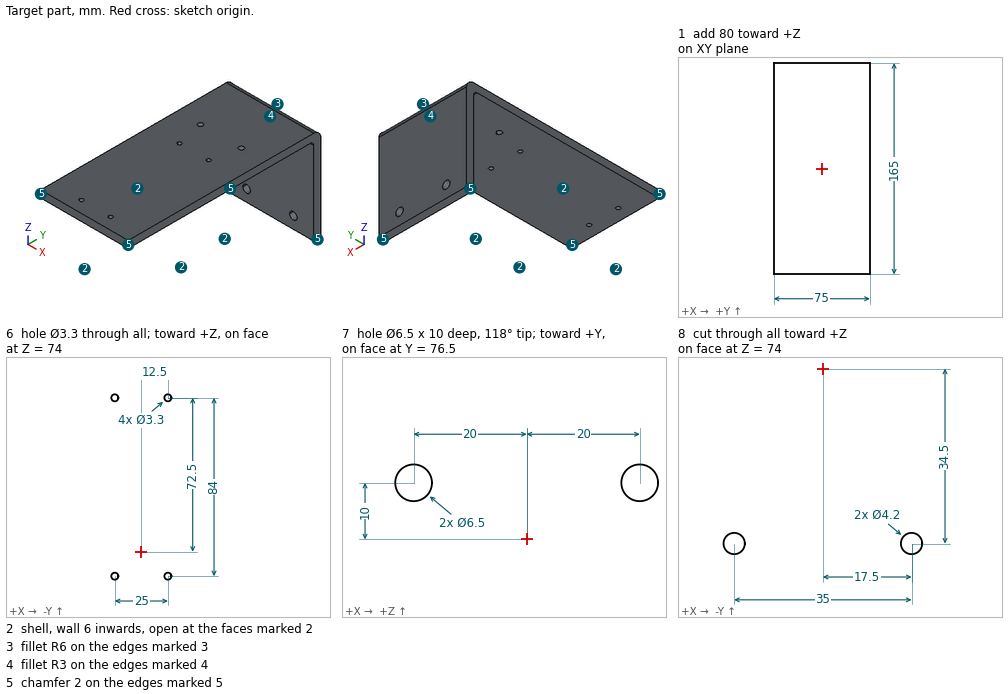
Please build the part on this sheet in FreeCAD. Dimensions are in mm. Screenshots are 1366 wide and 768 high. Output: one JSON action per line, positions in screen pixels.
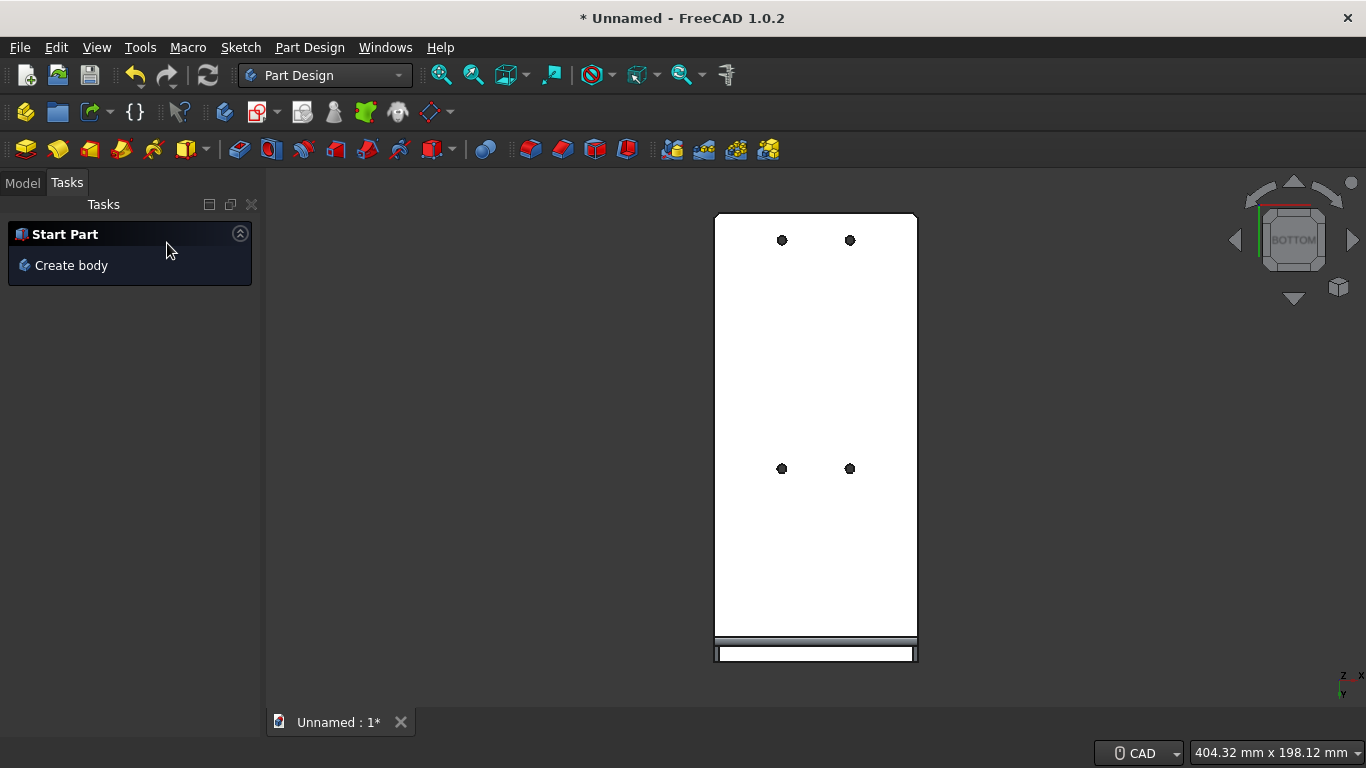
{"action": "left_click", "coordinate": [816, 364]}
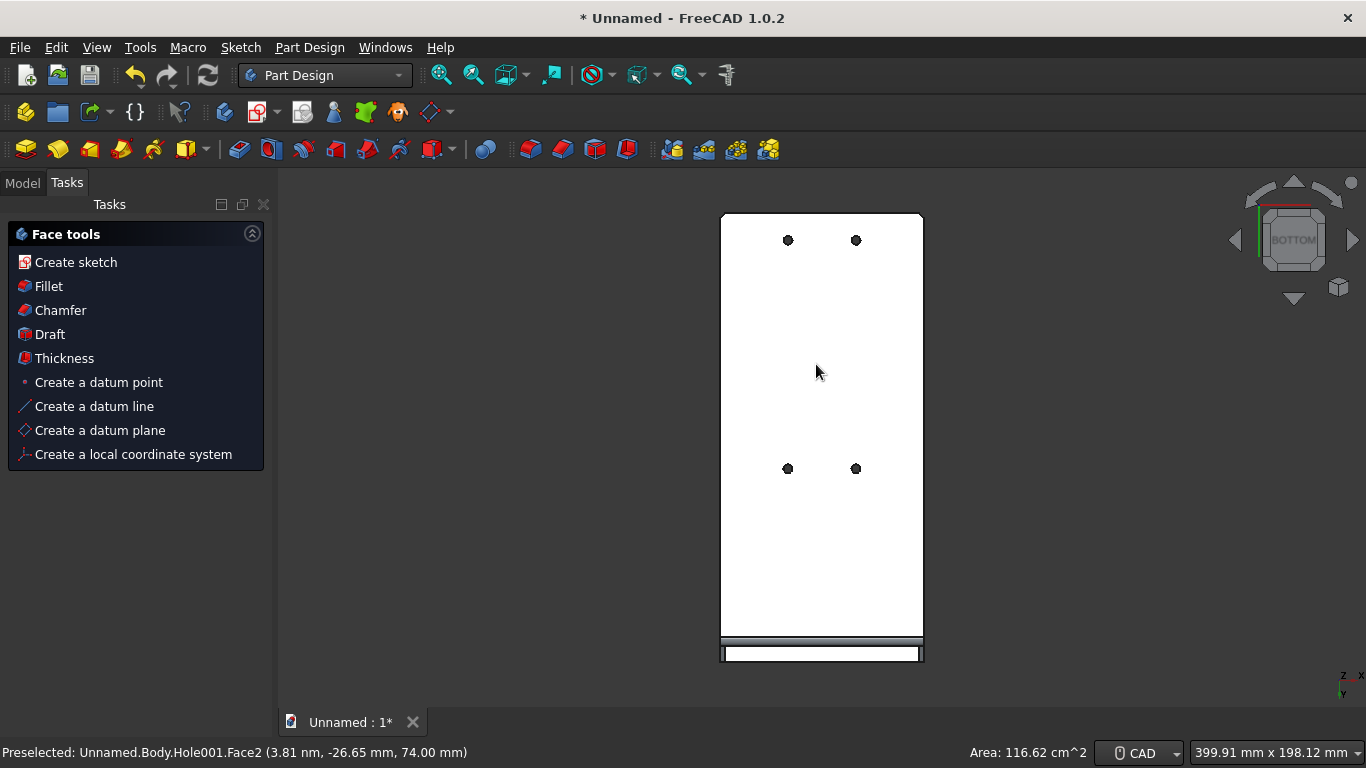
{"action": "left_click", "coordinate": [258, 112]}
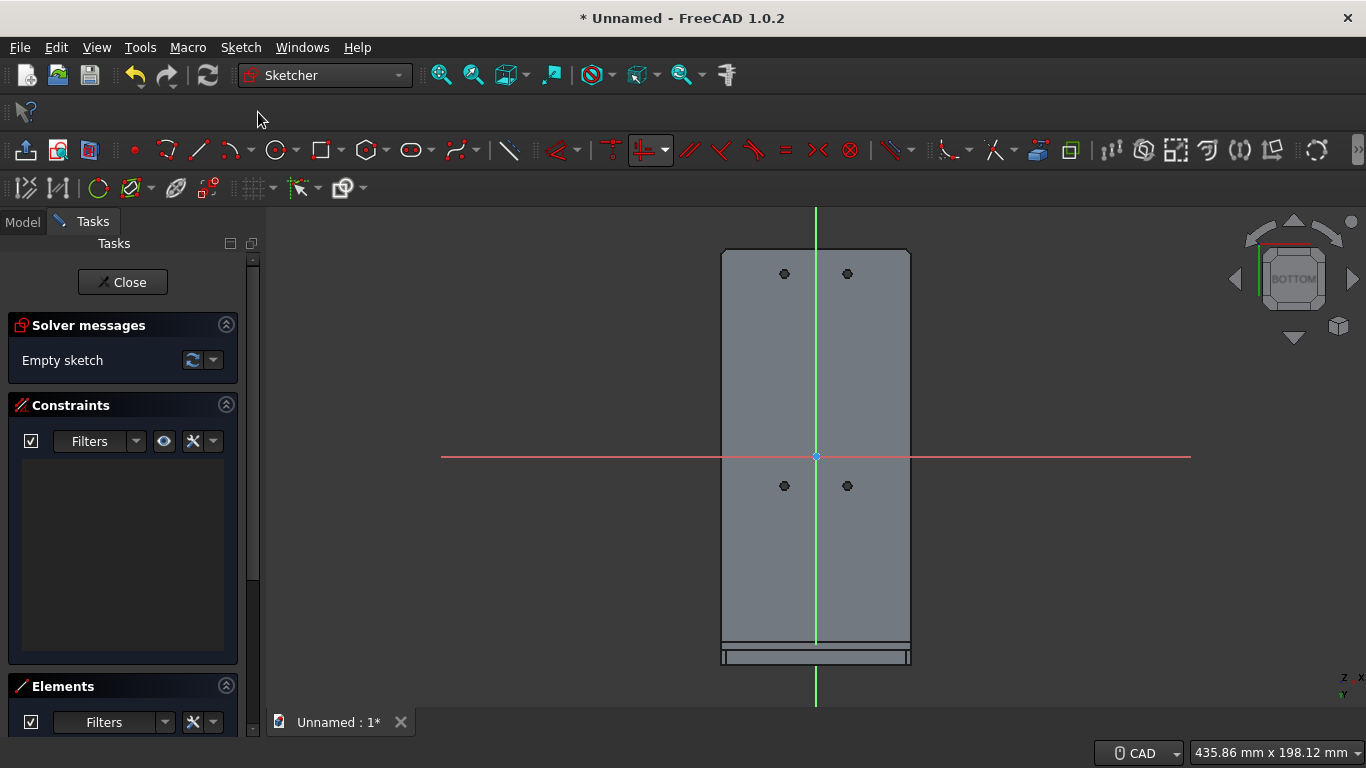
{"action": "left_click", "coordinate": [90, 150]}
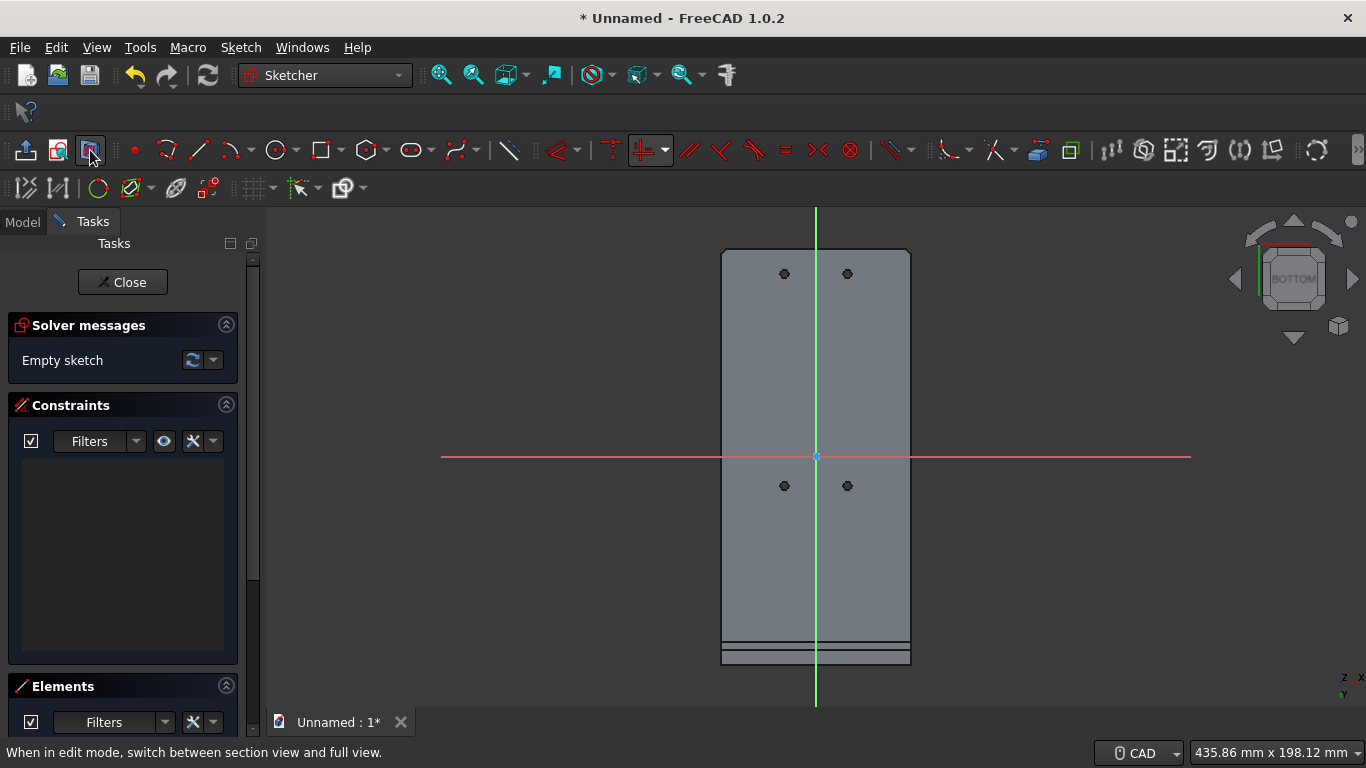
{"action": "scroll", "coordinate": [846, 523], "scroll_direction": "up", "scroll_amount": 6}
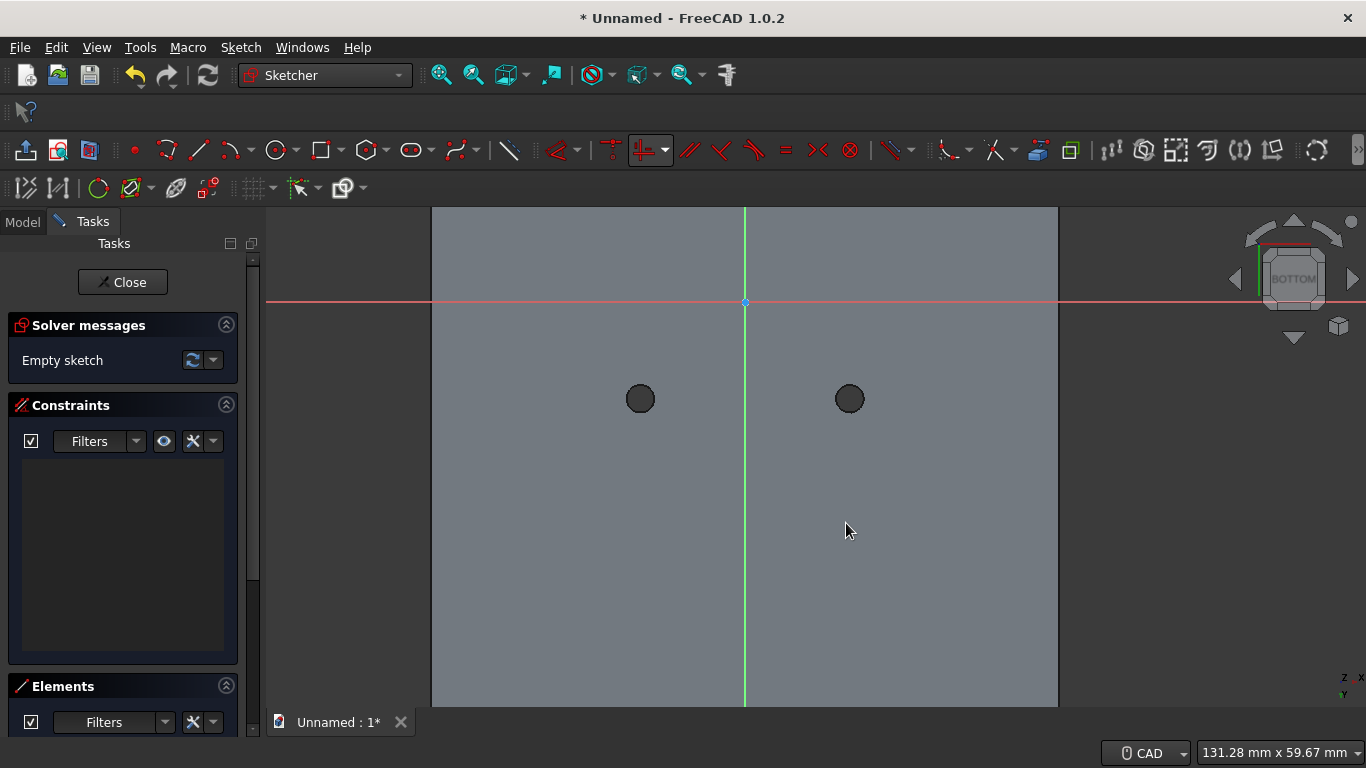
{"action": "left_click", "coordinate": [276, 150]}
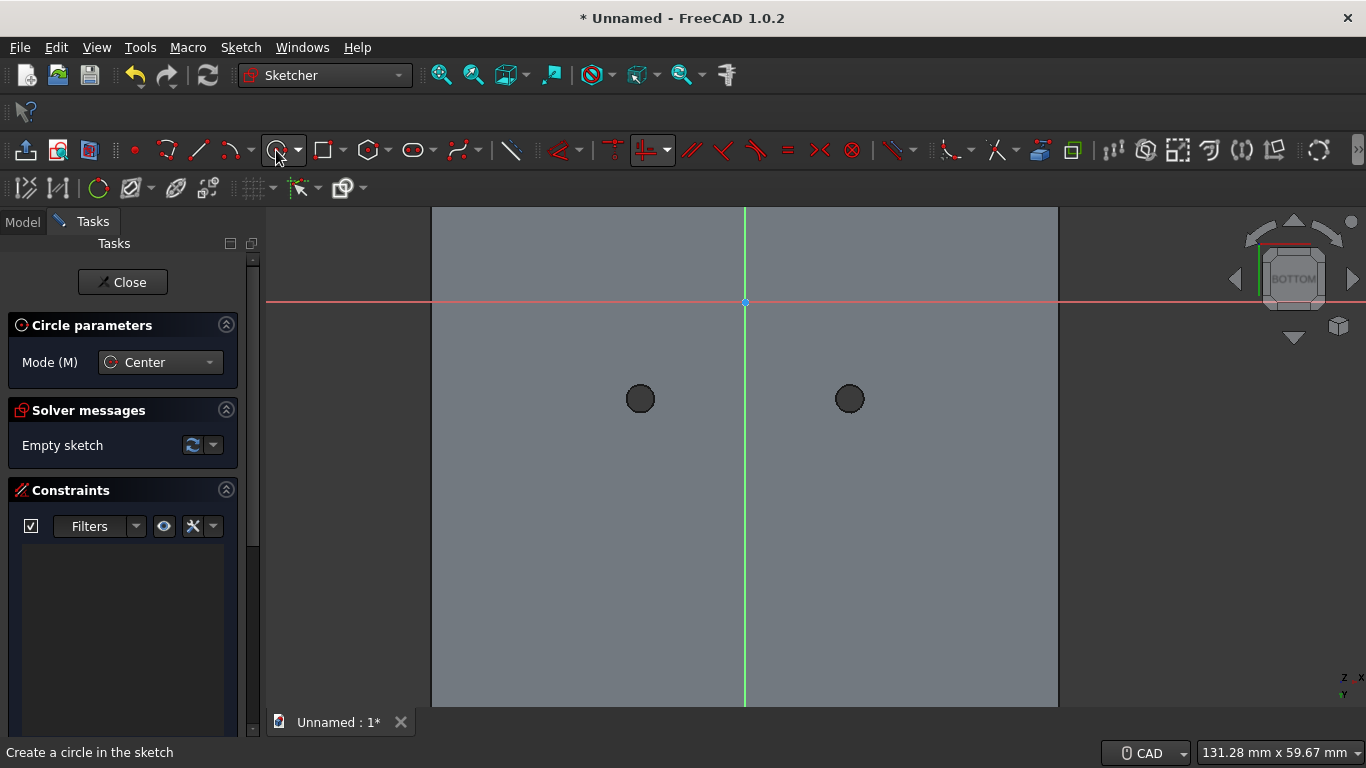
{"action": "scroll", "coordinate": [892, 591], "scroll_direction": "up", "scroll_amount": 2}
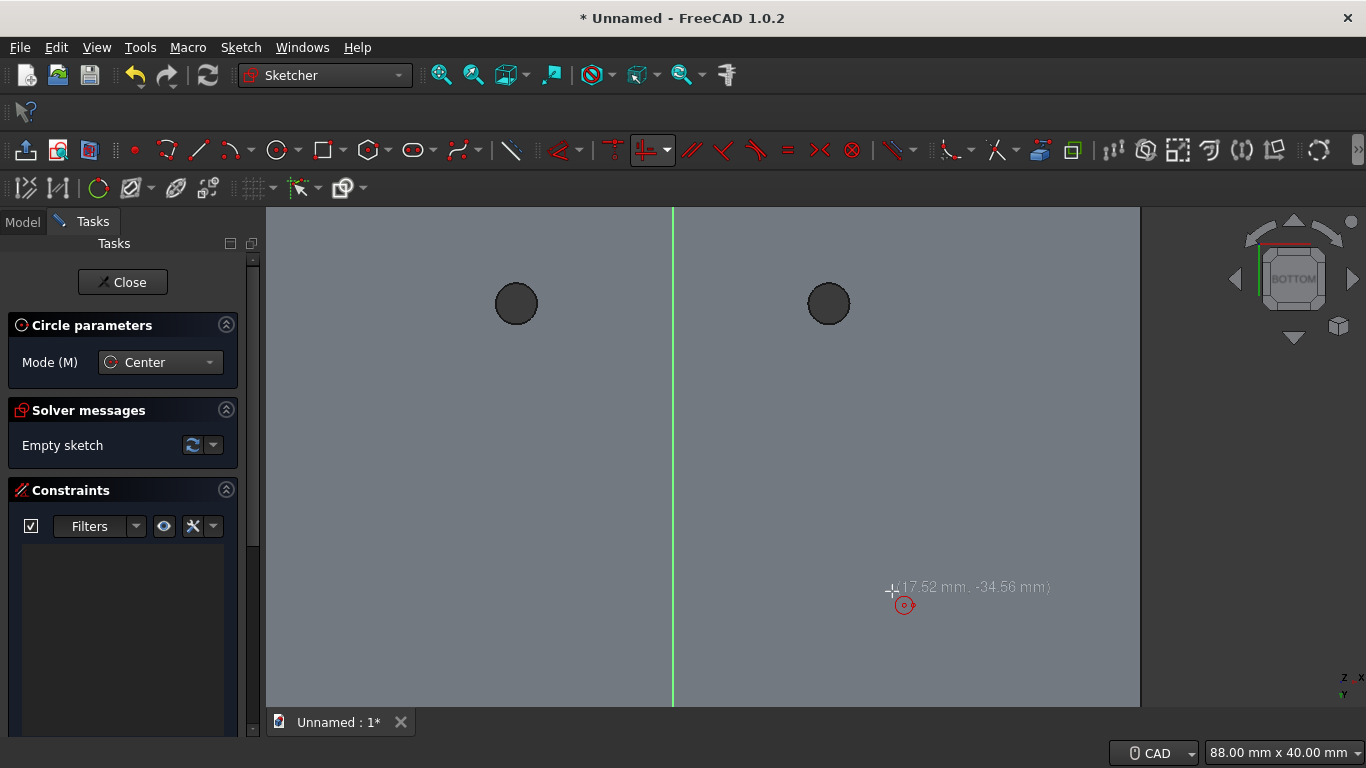
{"action": "left_click", "coordinate": [891, 591]}
{"action": "left_click", "coordinate": [910, 573]}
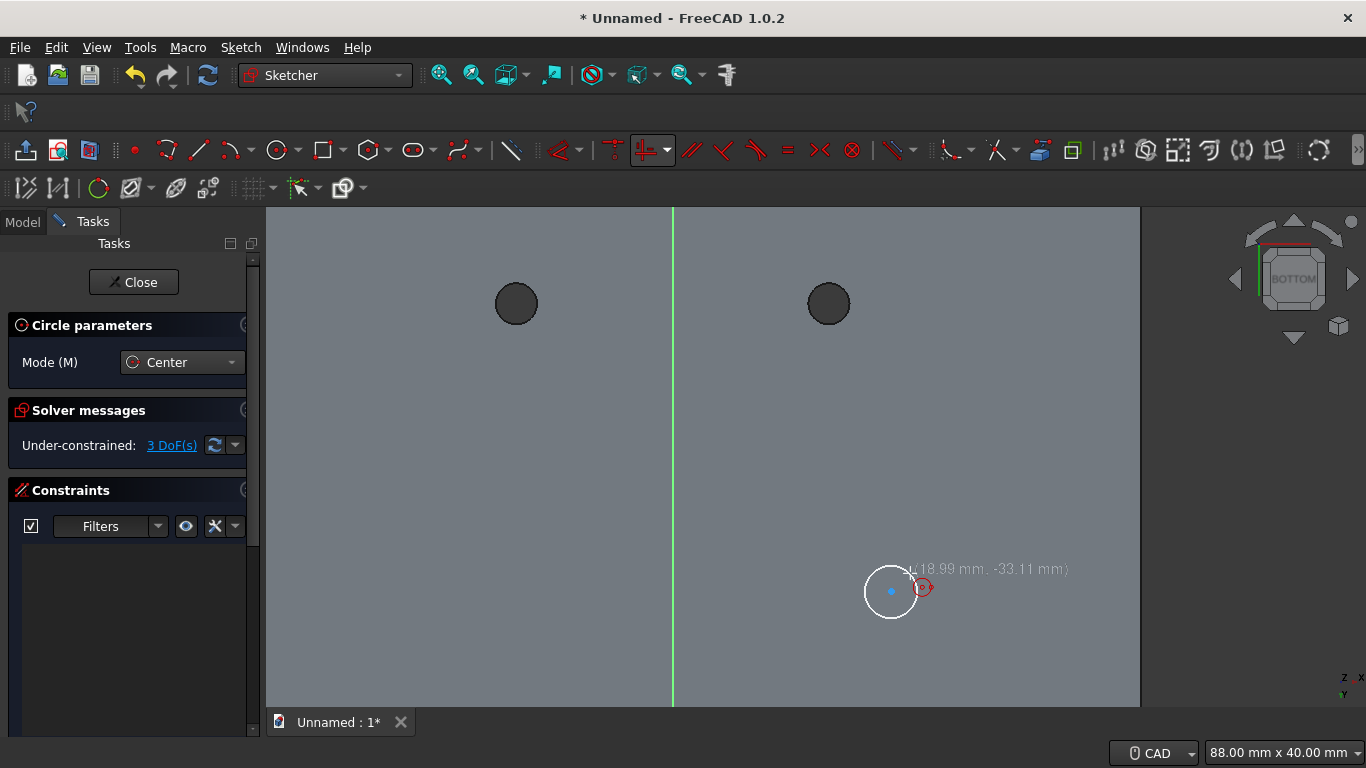
{"action": "left_click", "coordinate": [454, 591]}
{"action": "left_click", "coordinate": [472, 573]}
{"action": "key", "text": "Escape"}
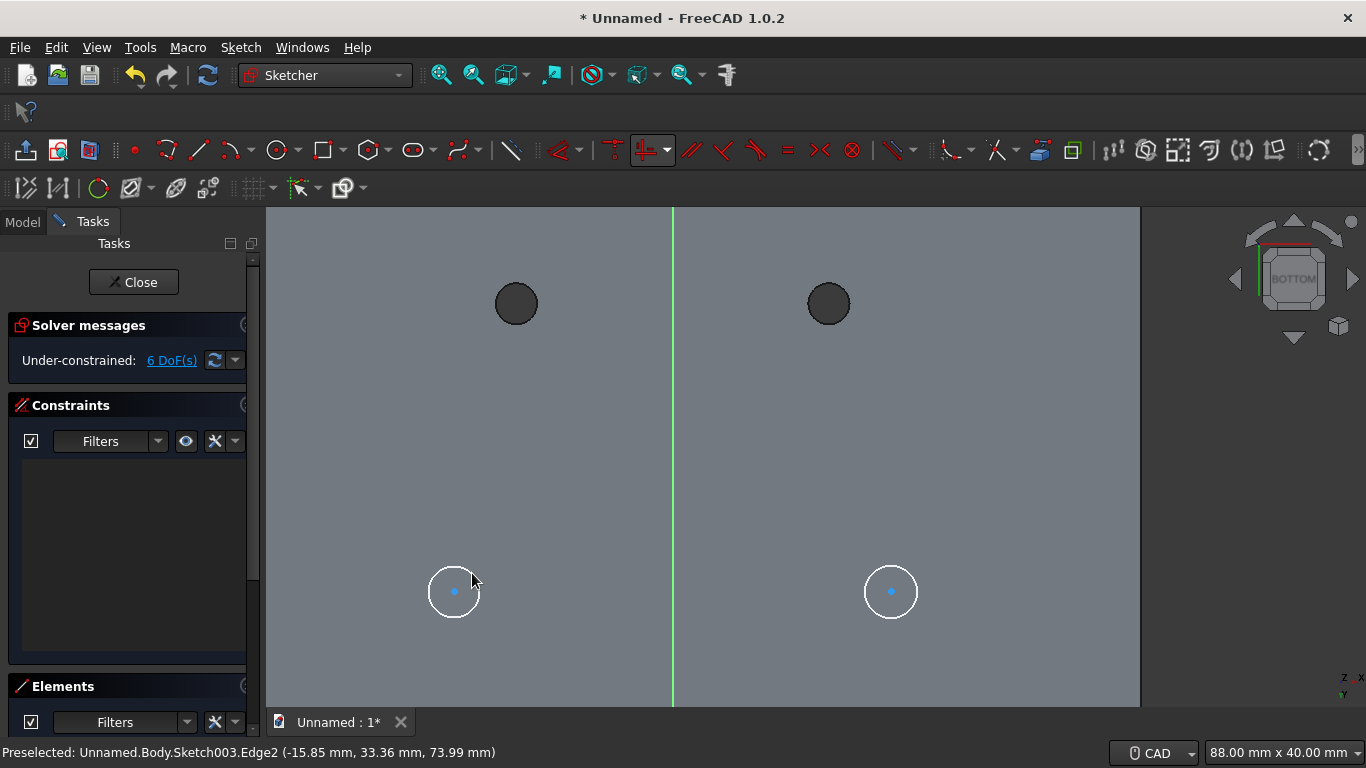
{"action": "left_click", "coordinate": [909, 573]}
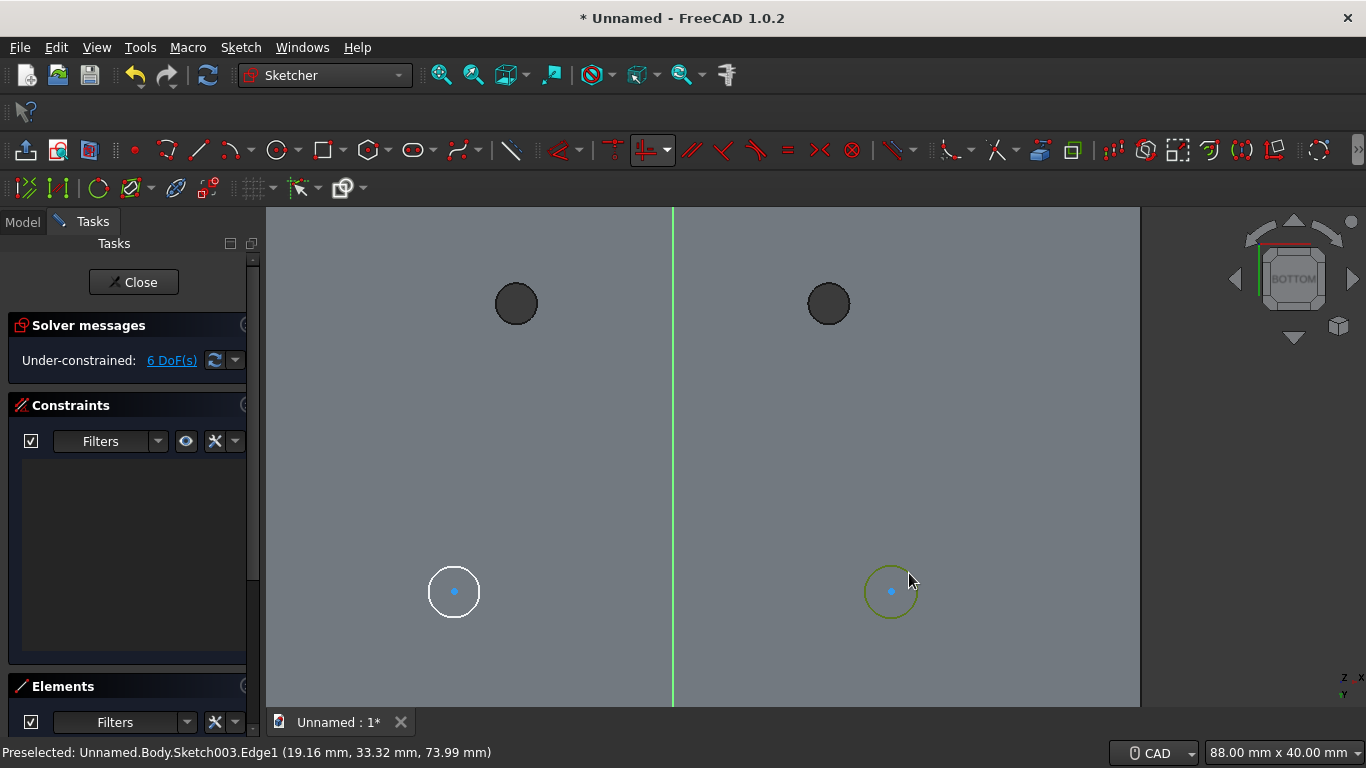
{"action": "left_click", "coordinate": [472, 574]}